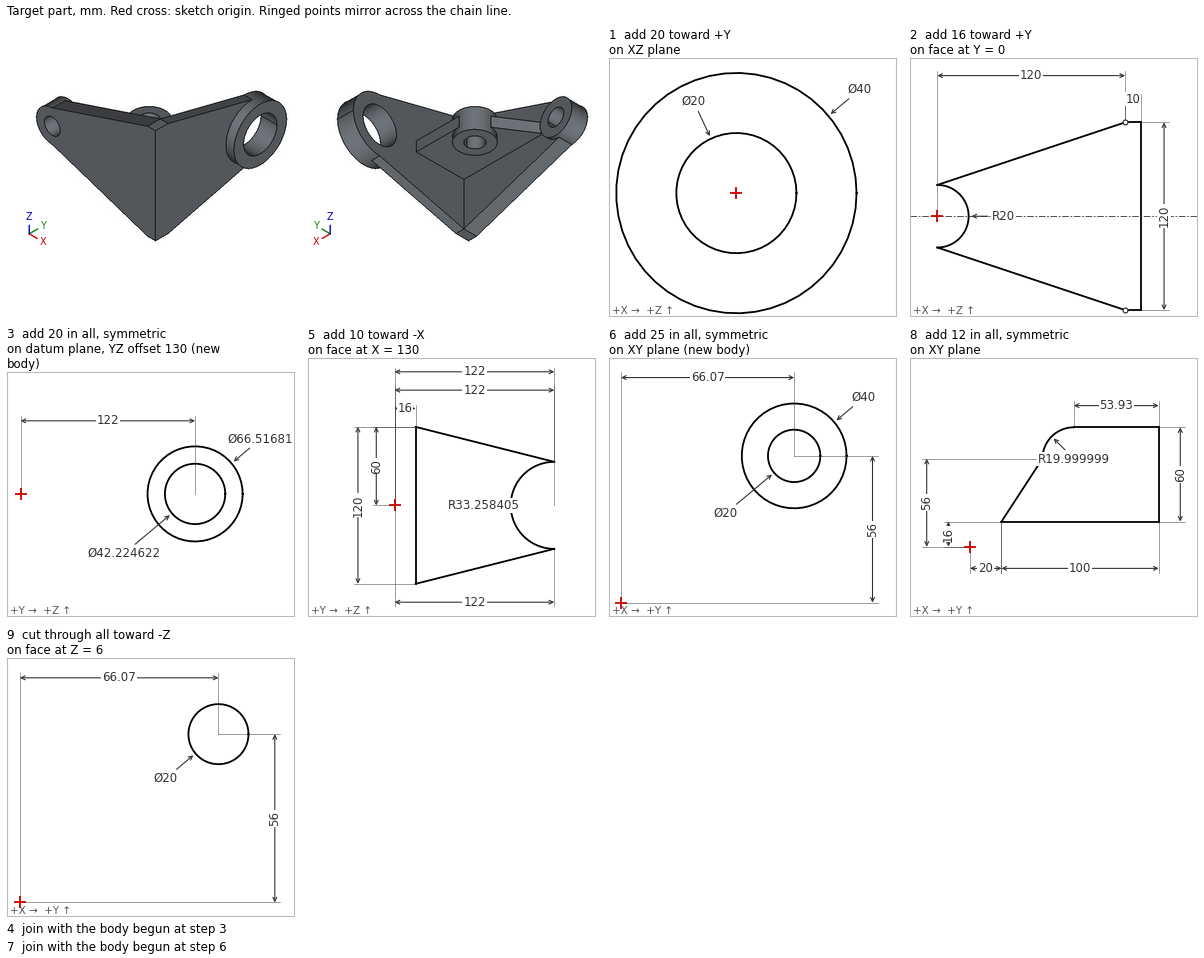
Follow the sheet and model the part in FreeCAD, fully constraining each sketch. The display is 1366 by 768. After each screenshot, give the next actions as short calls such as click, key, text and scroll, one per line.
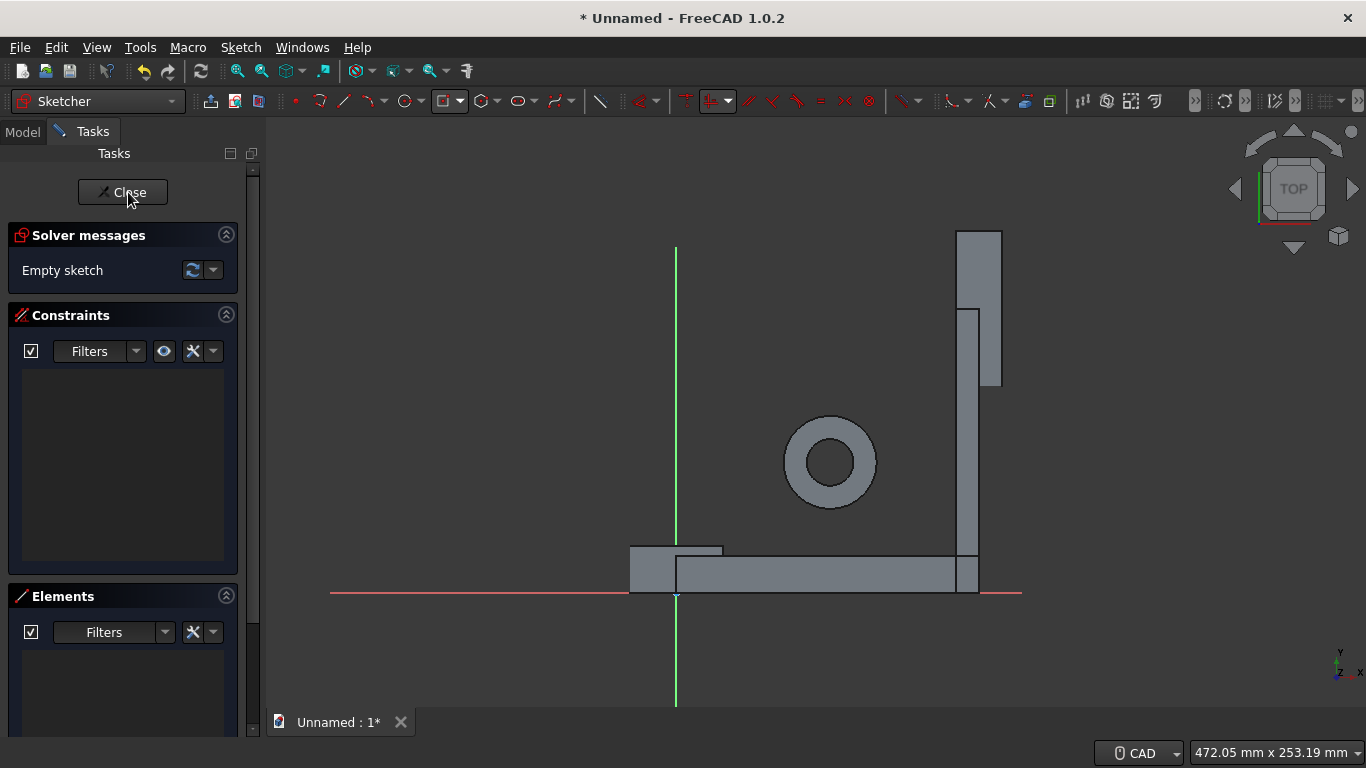
click(260, 102)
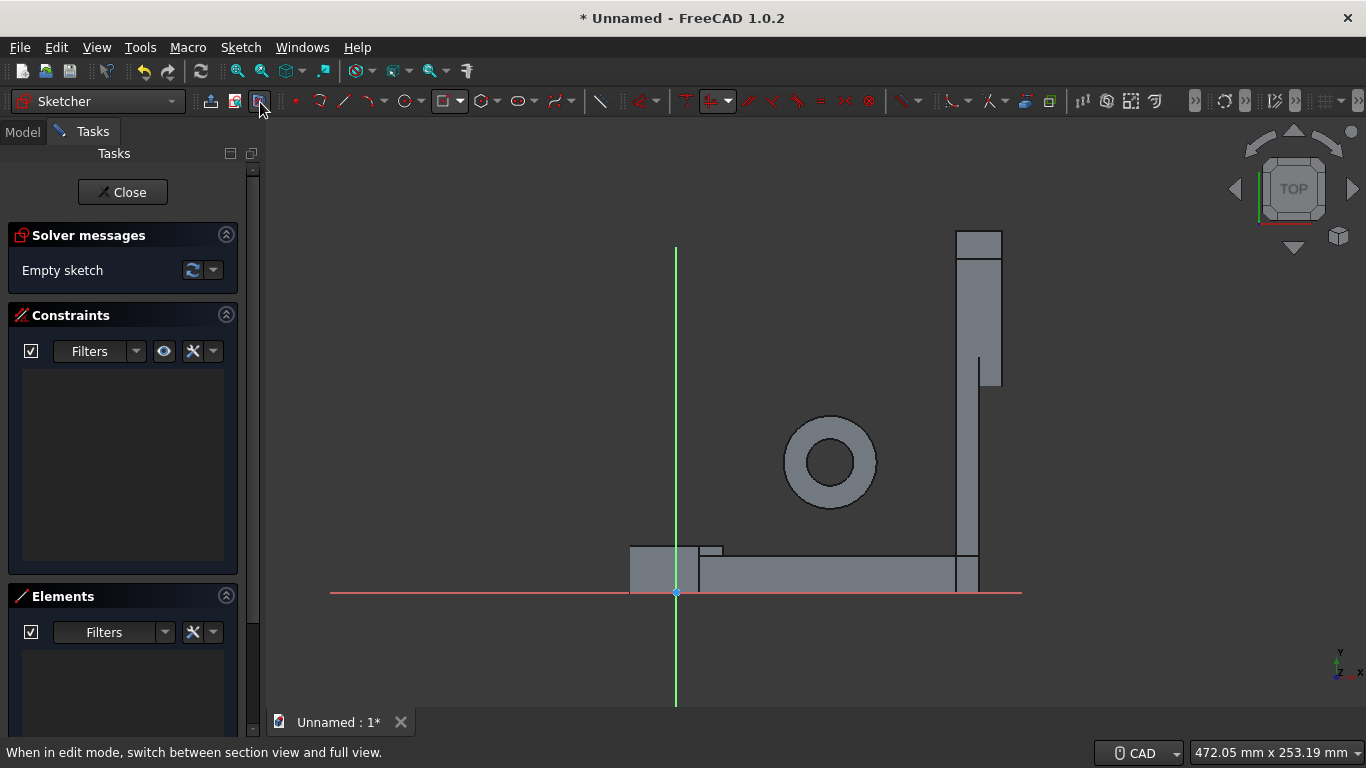
scroll(872, 580, up, 4)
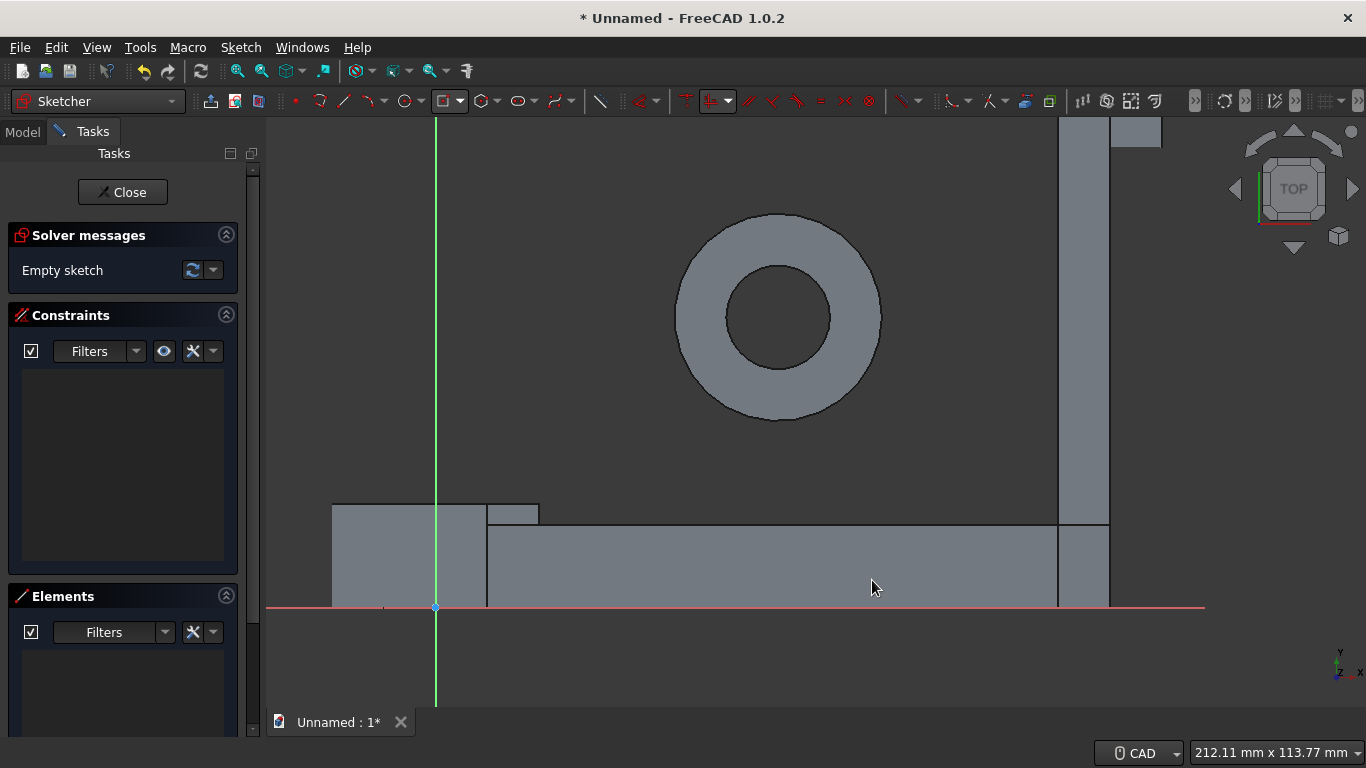
click(320, 102)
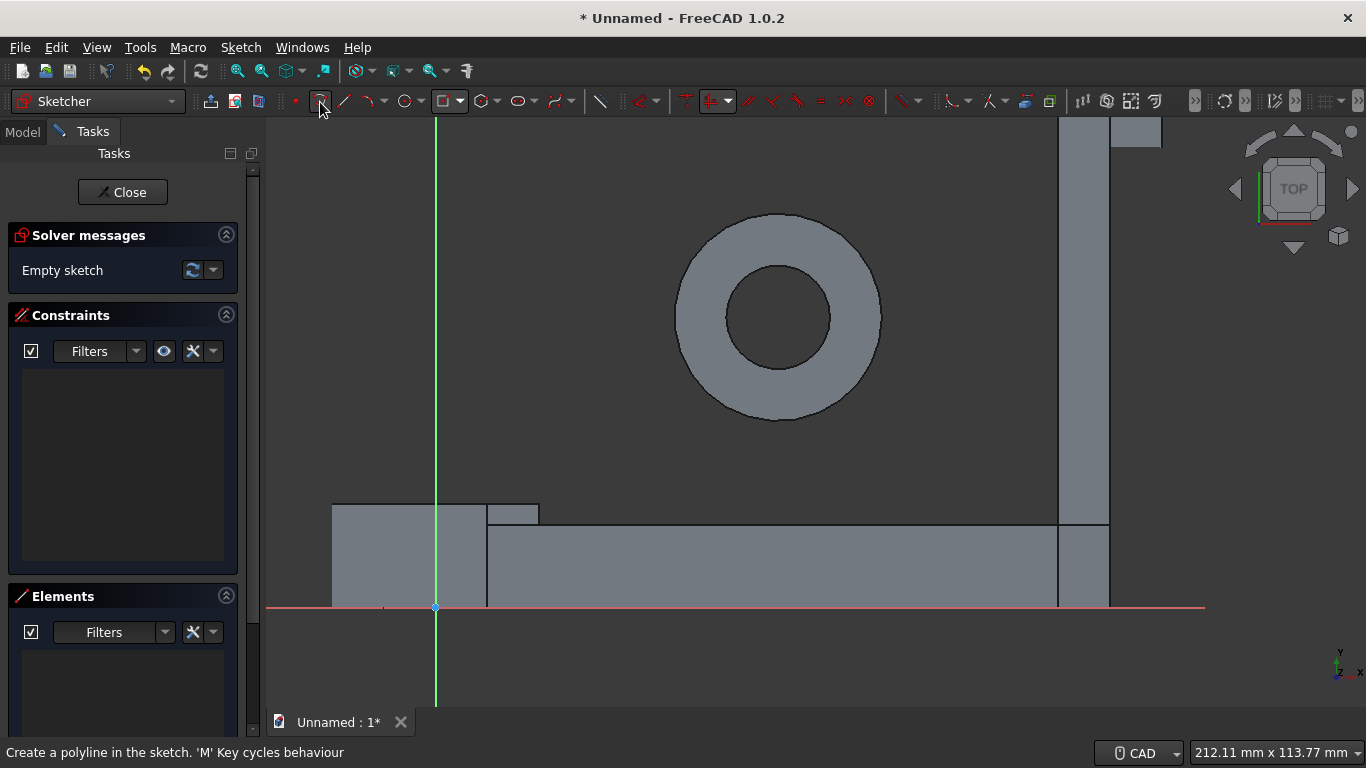
click(674, 317)
click(539, 525)
click(1058, 525)
click(1058, 214)
click(778, 214)
right_click(778, 214)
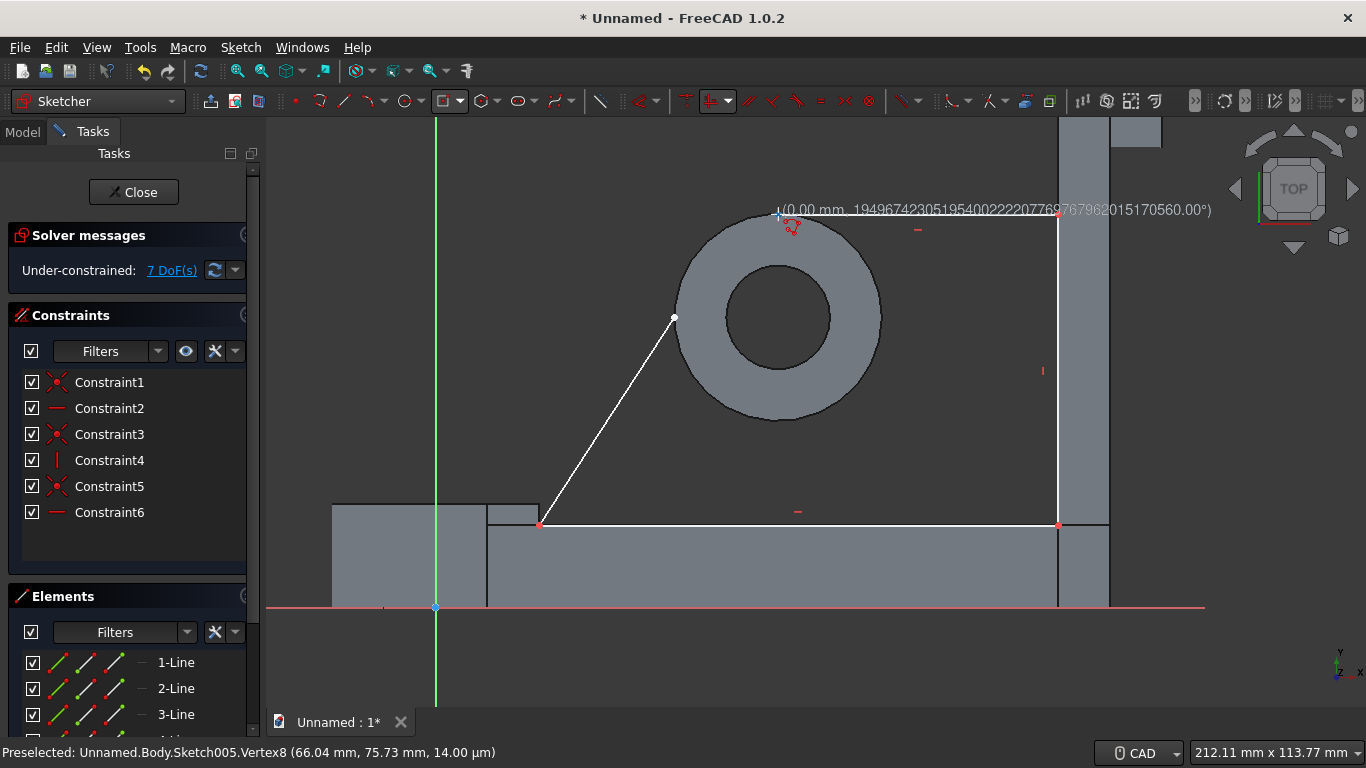
key(g)
key(3)
key(a)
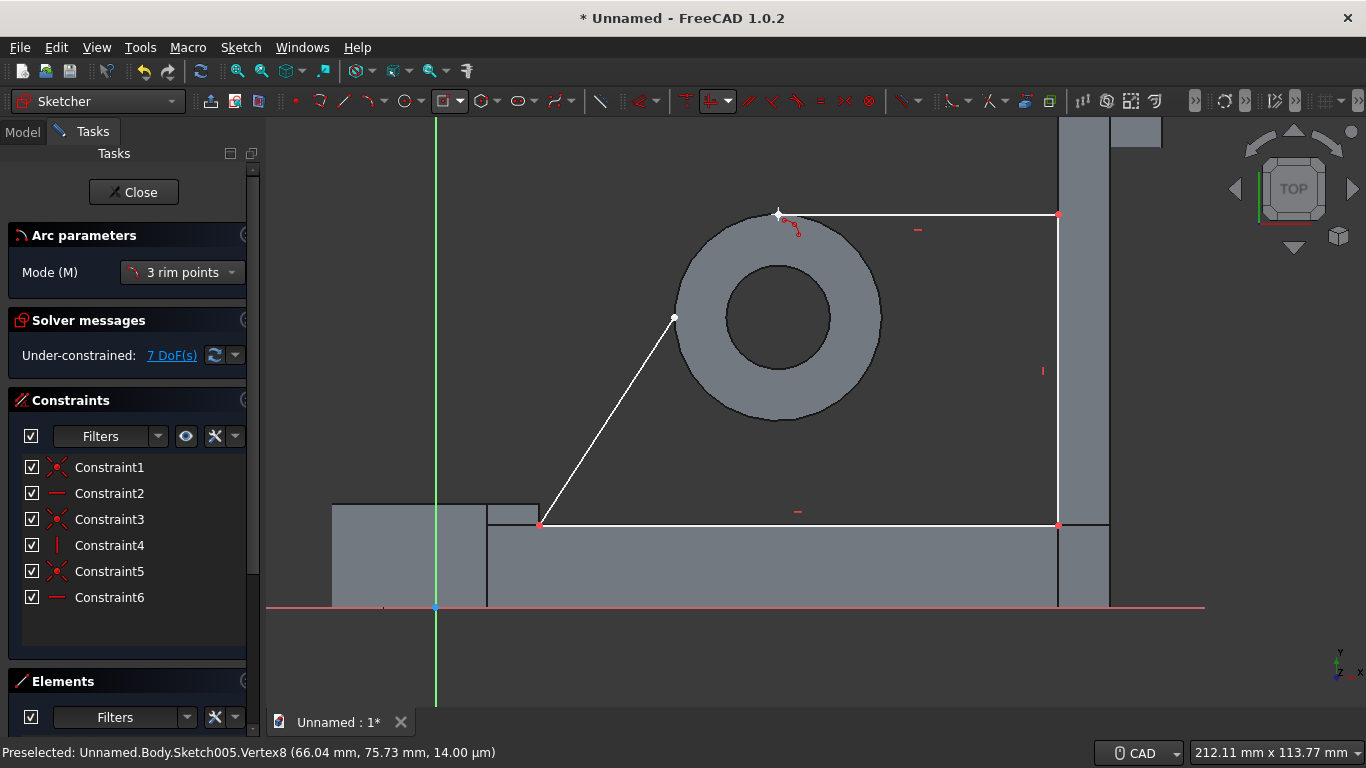
click(778, 215)
click(674, 318)
click(705, 244)
key(Escape)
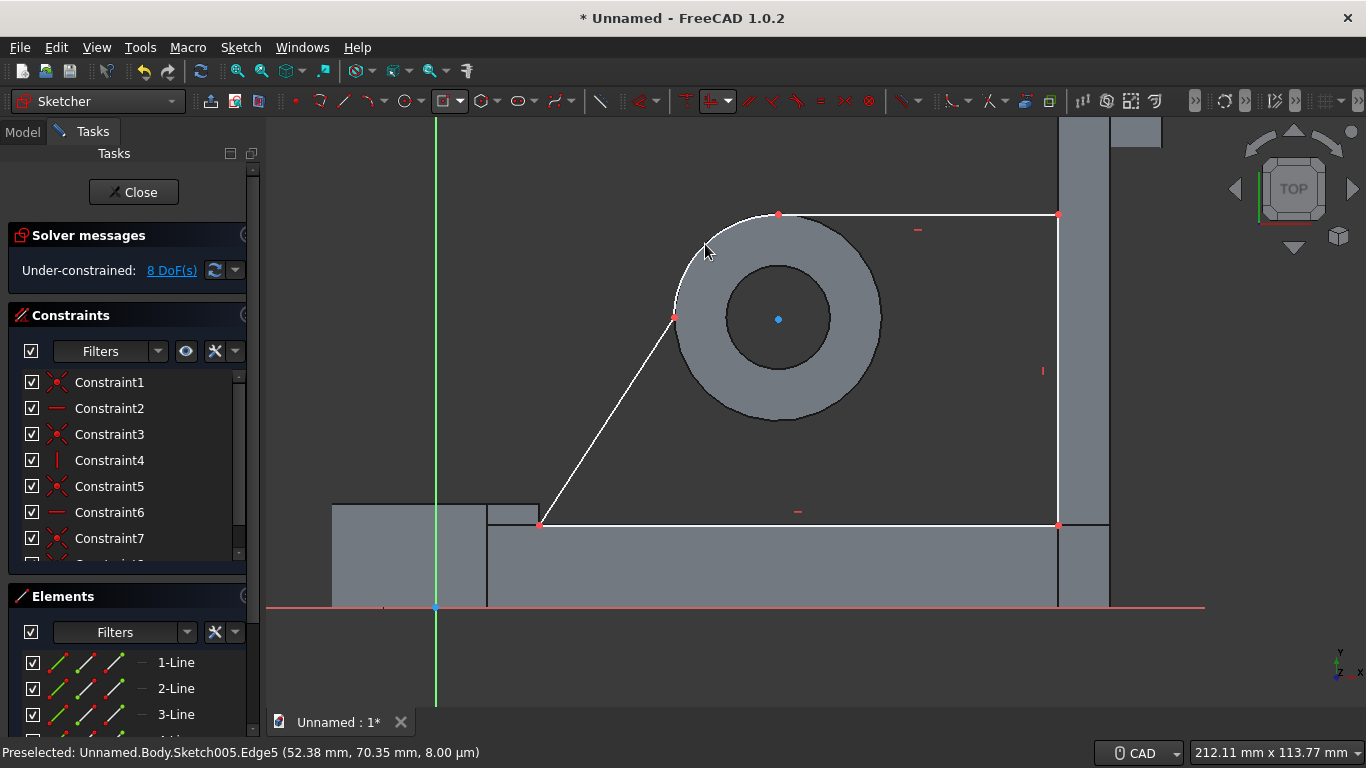
click(974, 215)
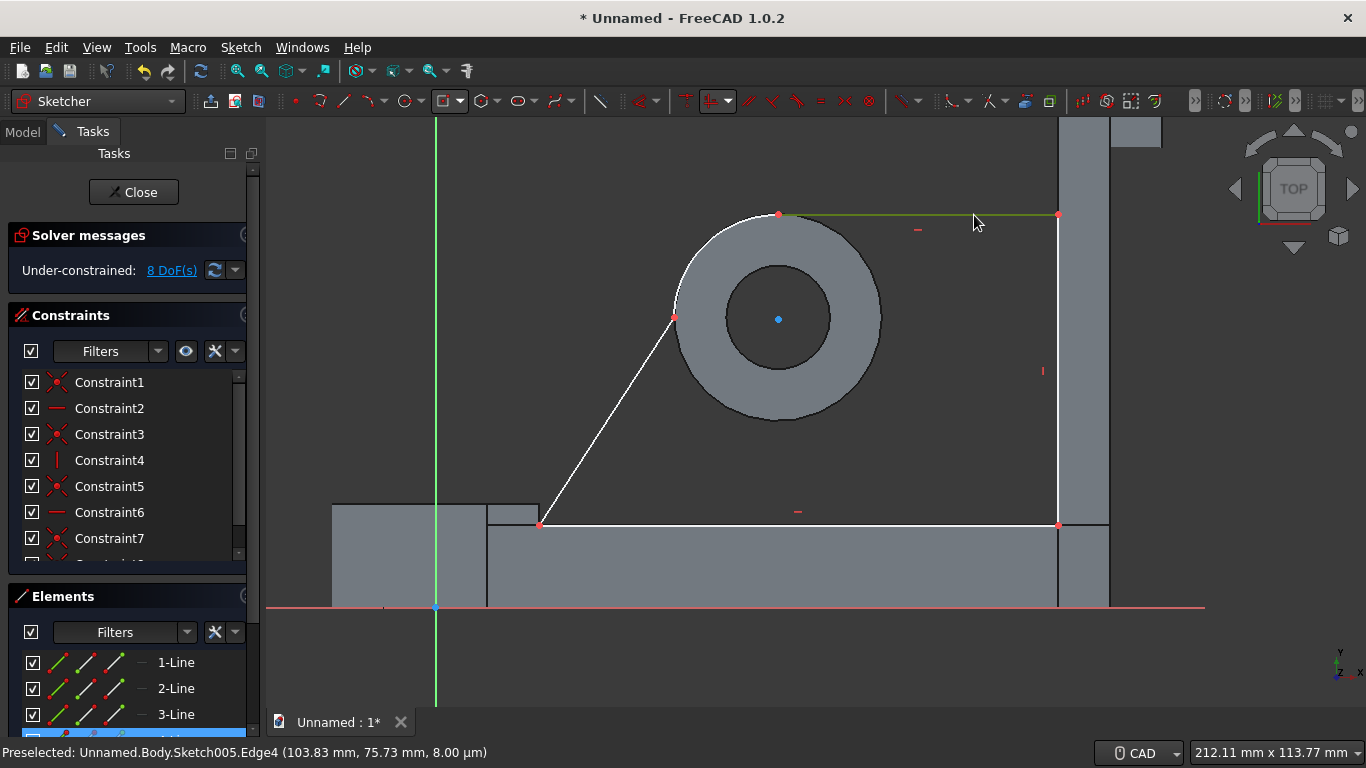
click(731, 226)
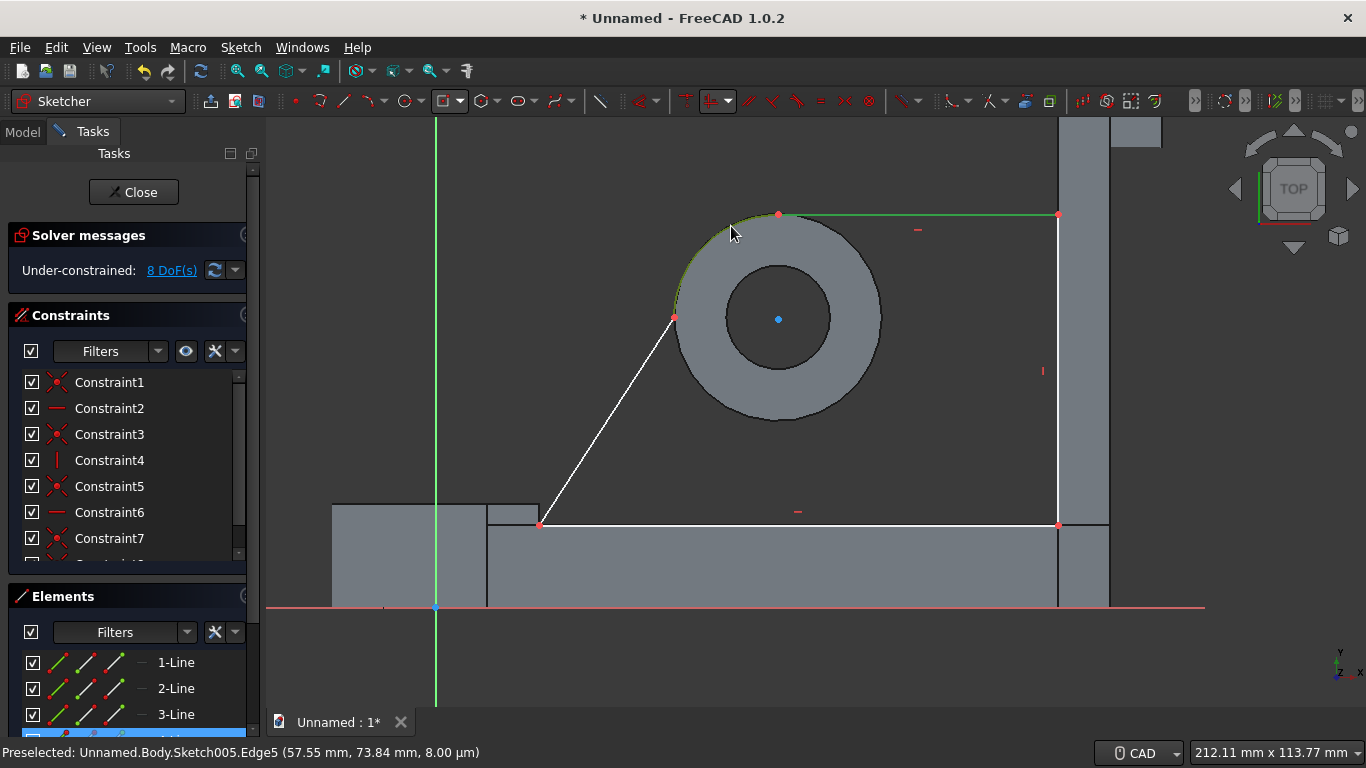
click(798, 102)